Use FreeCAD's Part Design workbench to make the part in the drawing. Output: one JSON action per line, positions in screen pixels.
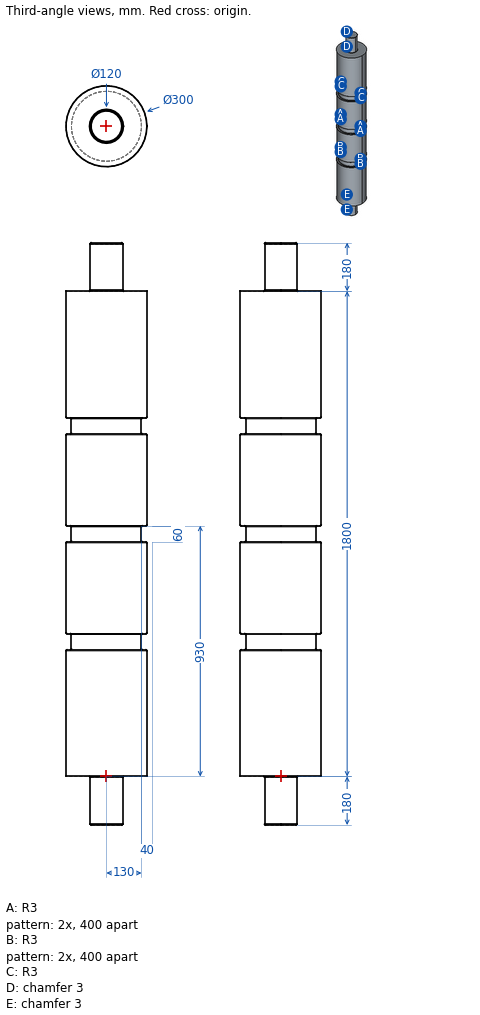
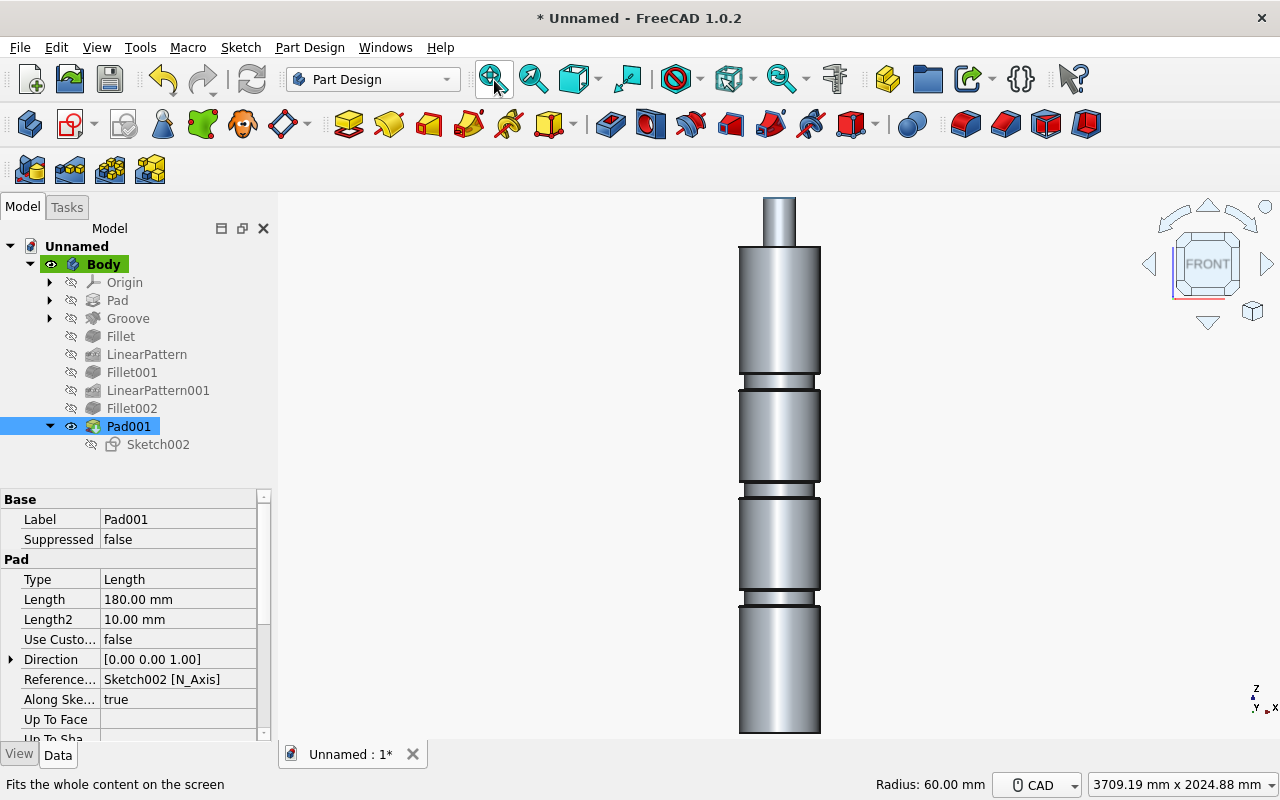
{"action": "key", "text": "3"}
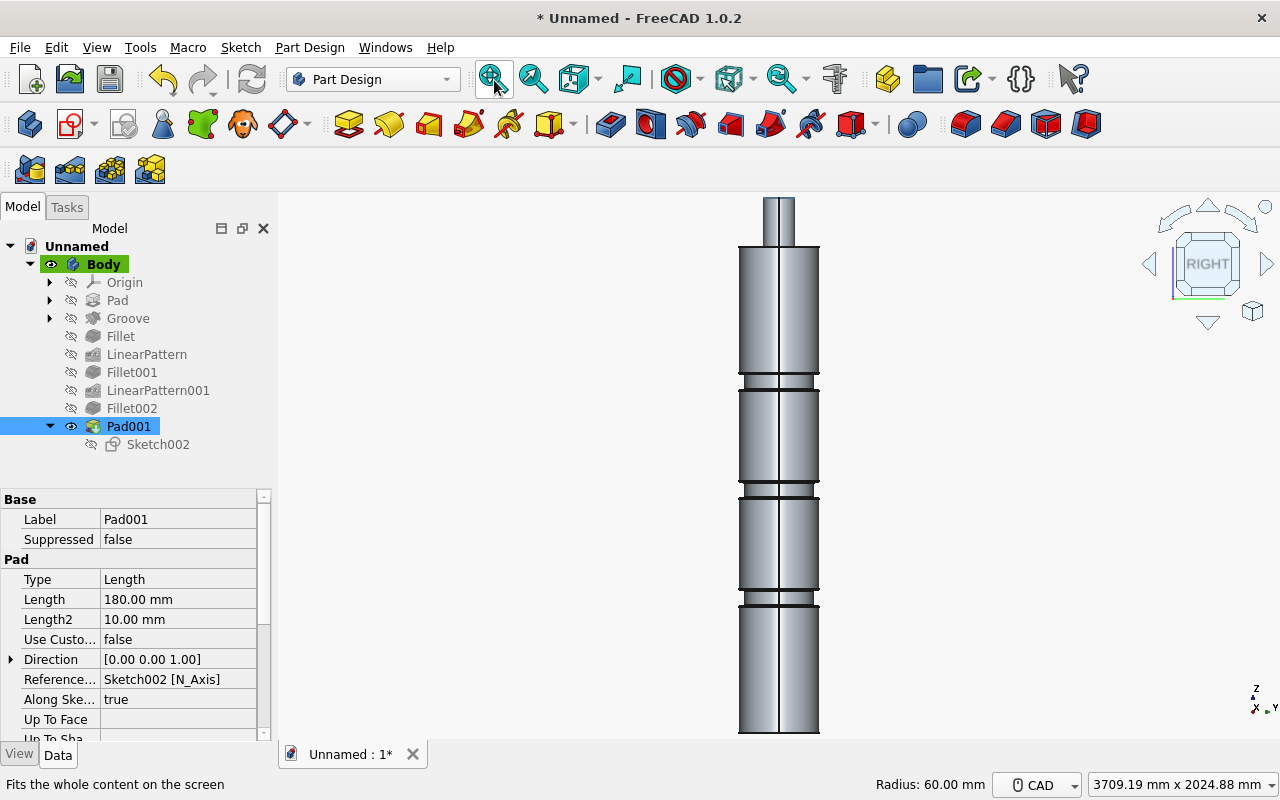
{"action": "key", "text": "5"}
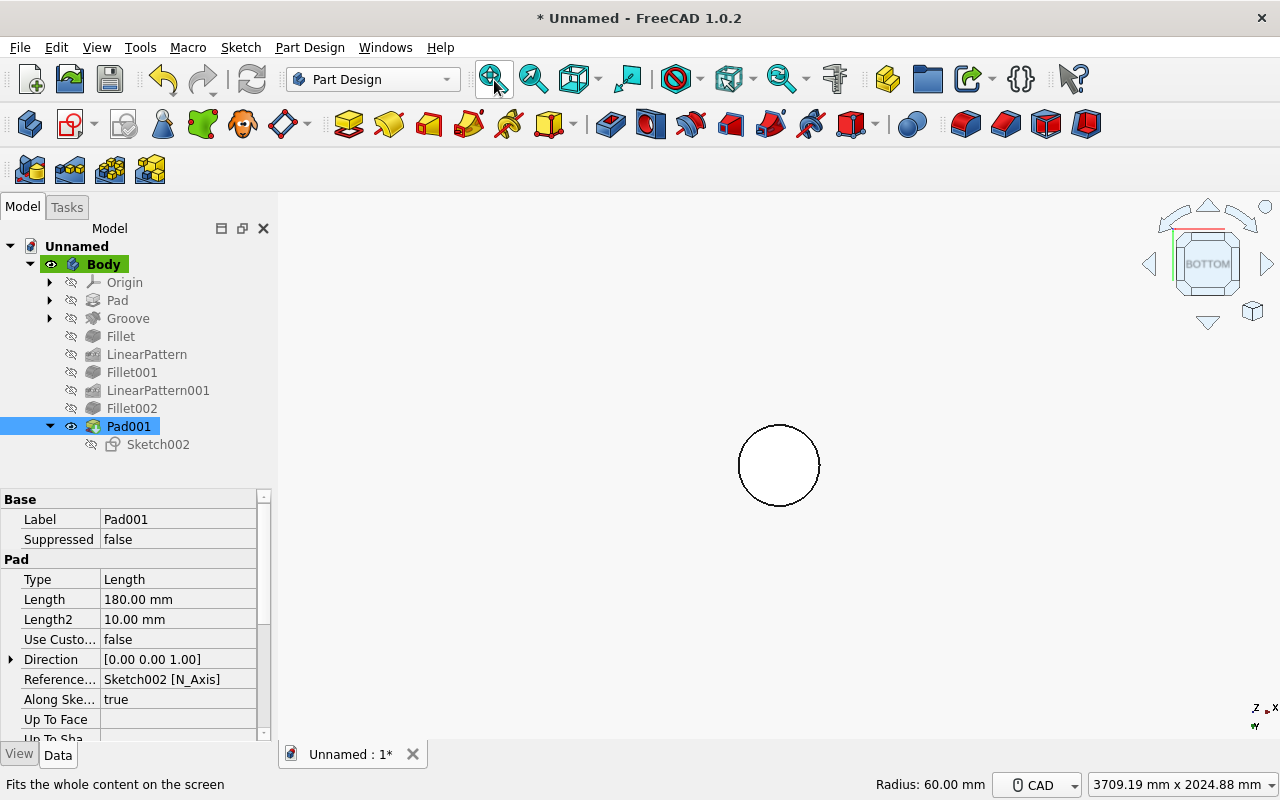
{"action": "left_click", "coordinate": [494, 80]}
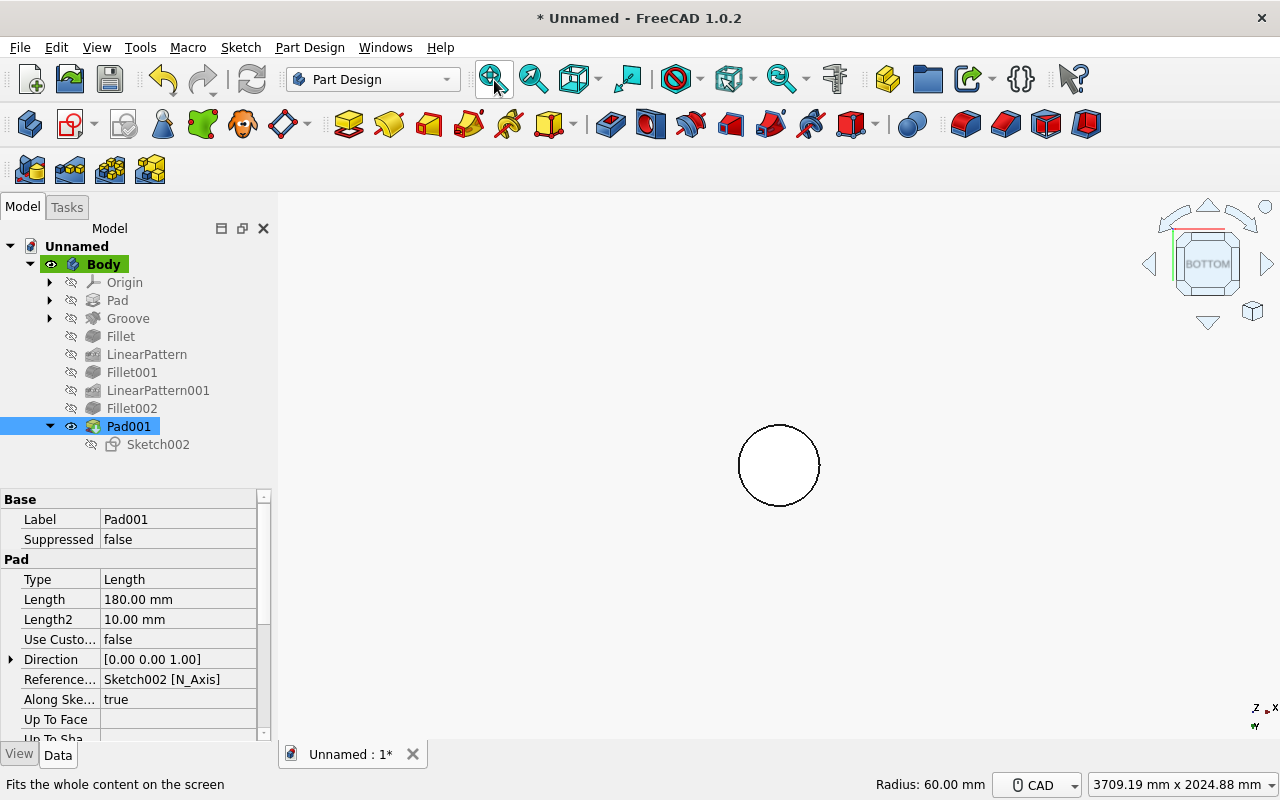
{"action": "key", "text": "4"}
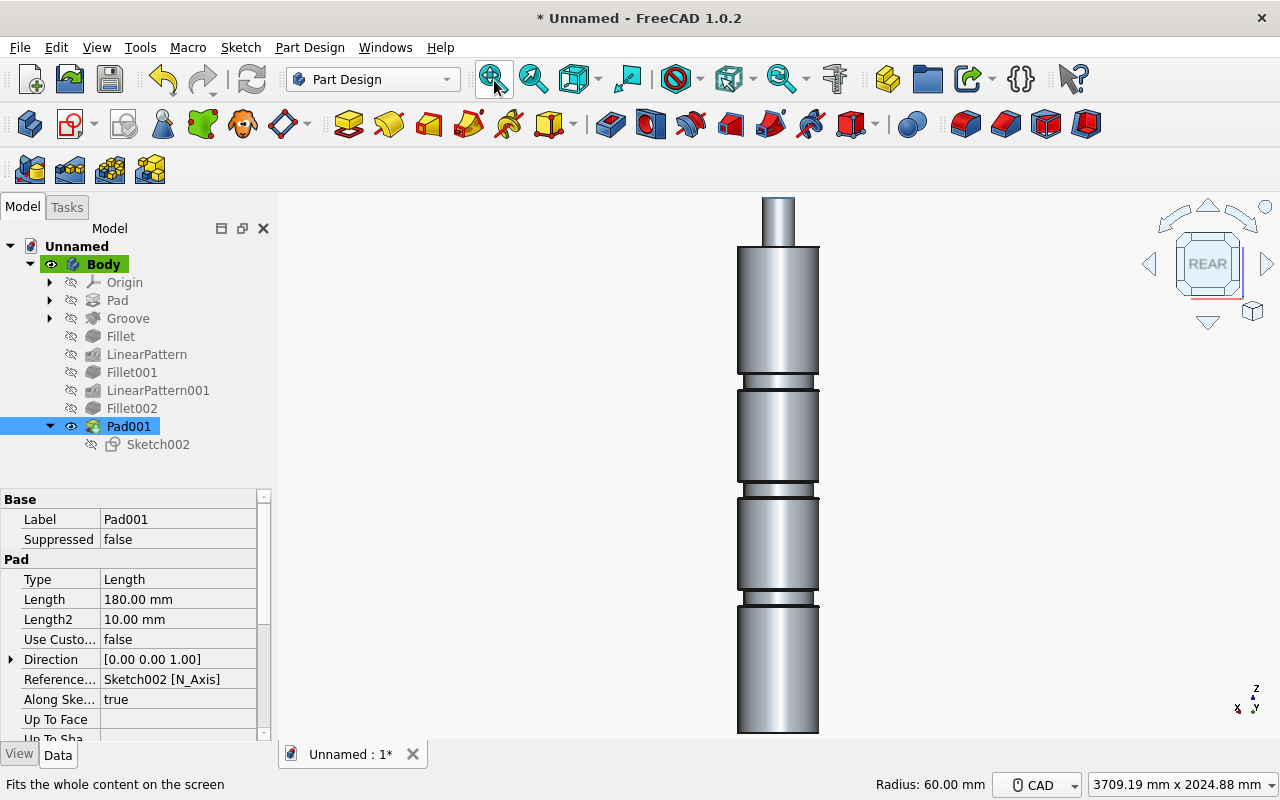
{"action": "key", "text": "6"}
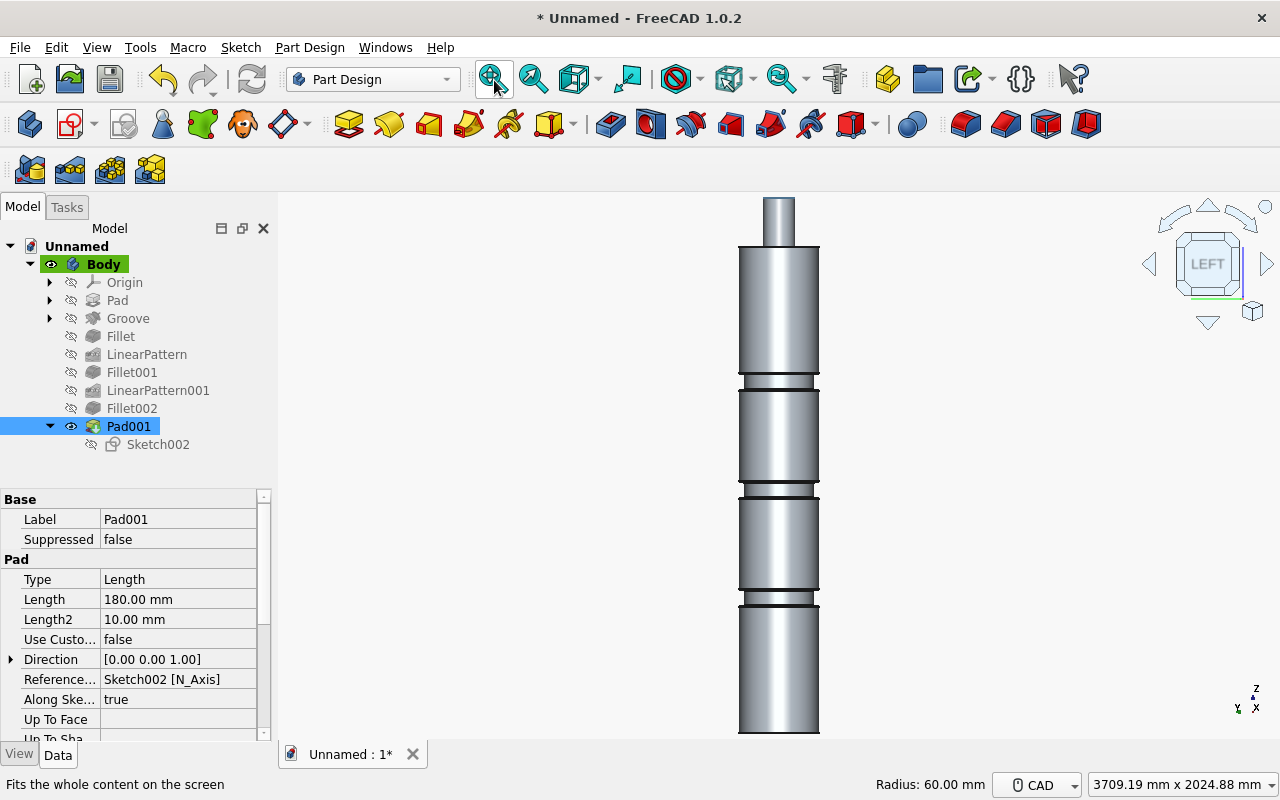
{"action": "key", "text": "v 3"}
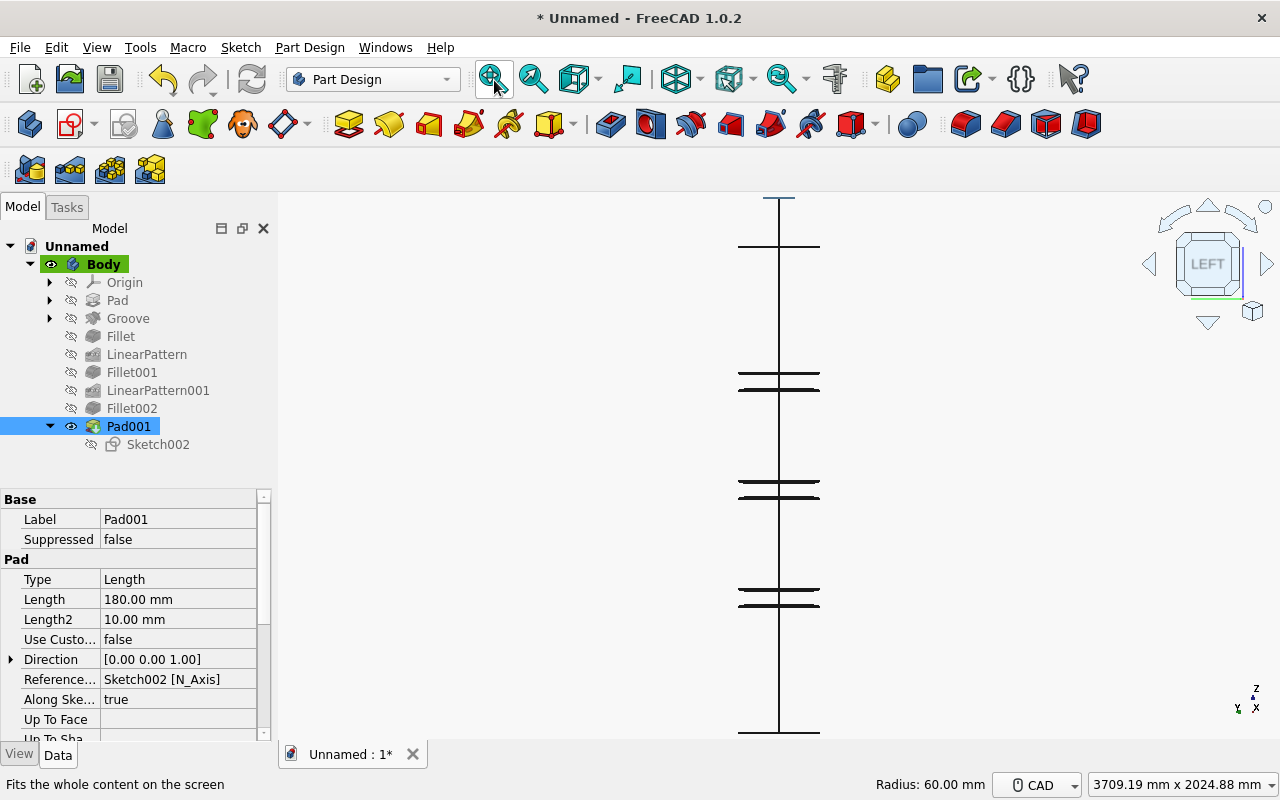
{"action": "key", "text": "0"}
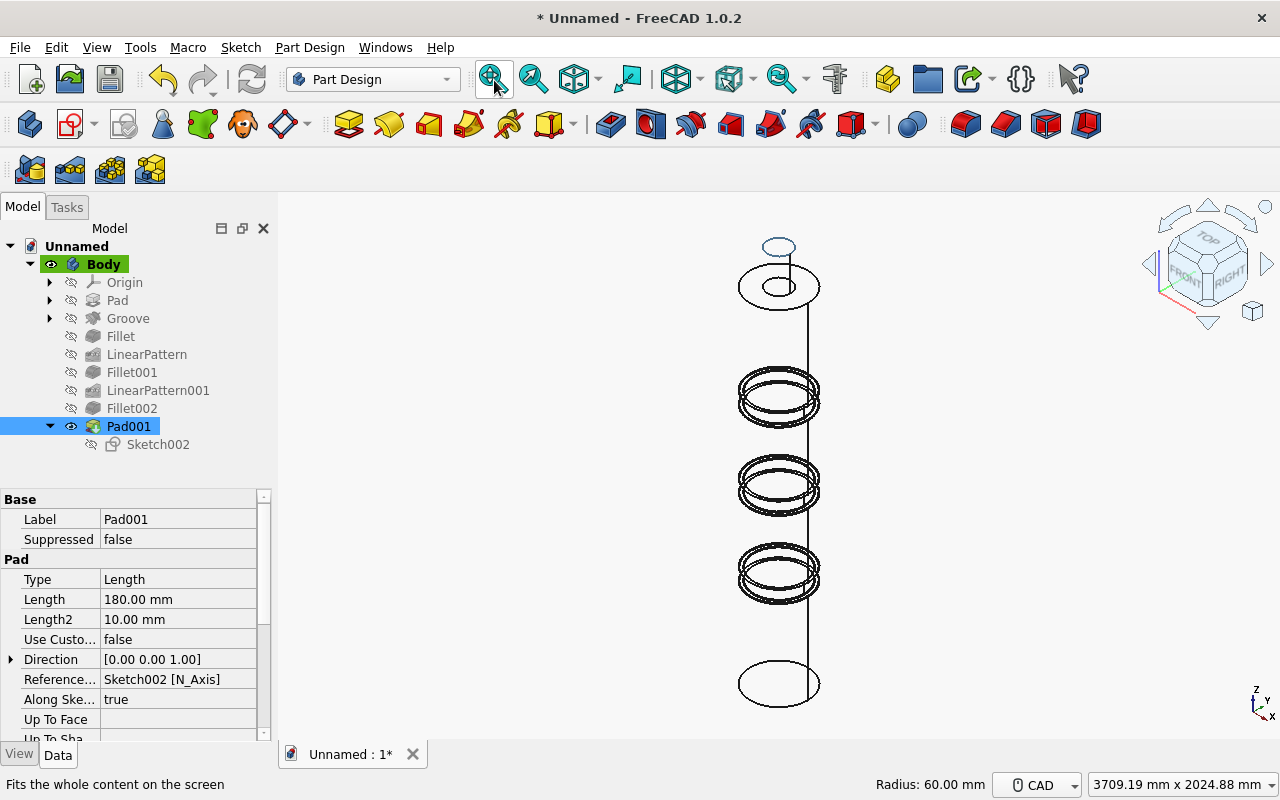
{"action": "left_click", "coordinate": [768, 279], "text": "ctrl"}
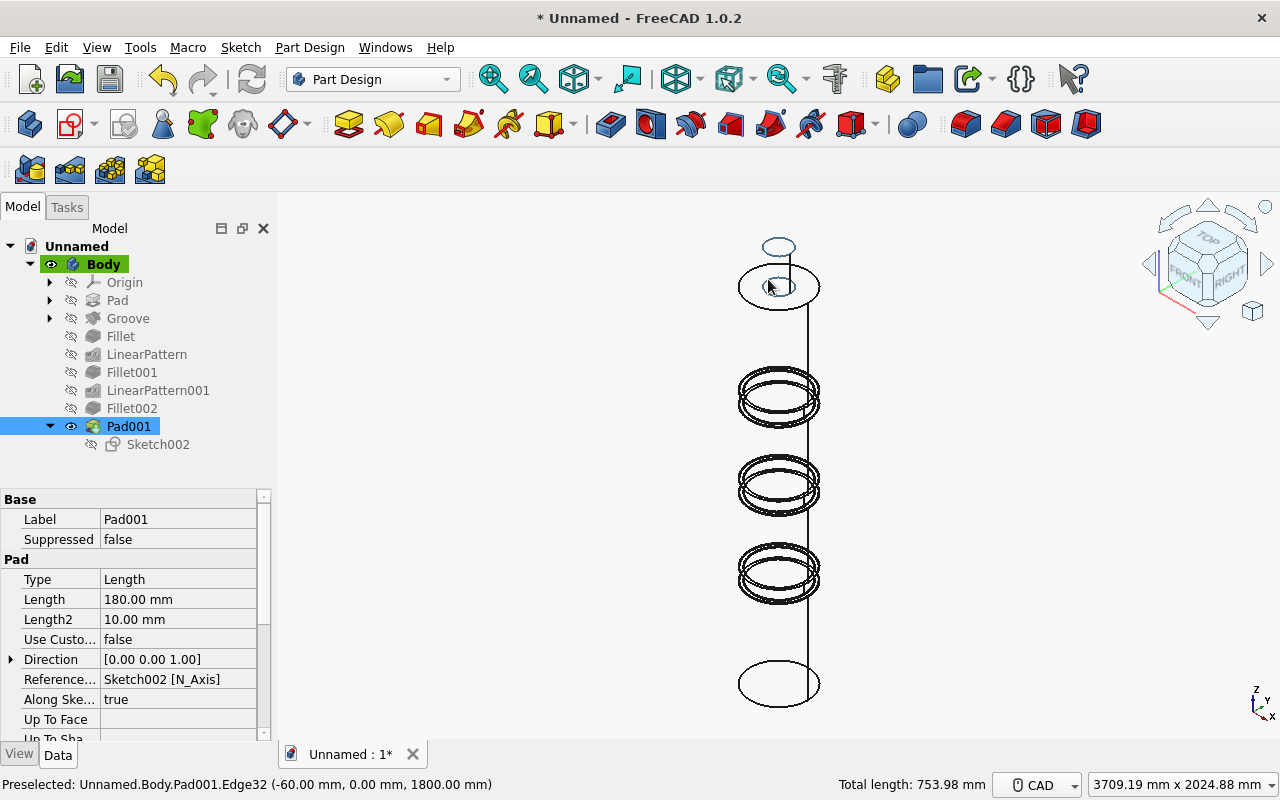
{"action": "key", "text": "v 1"}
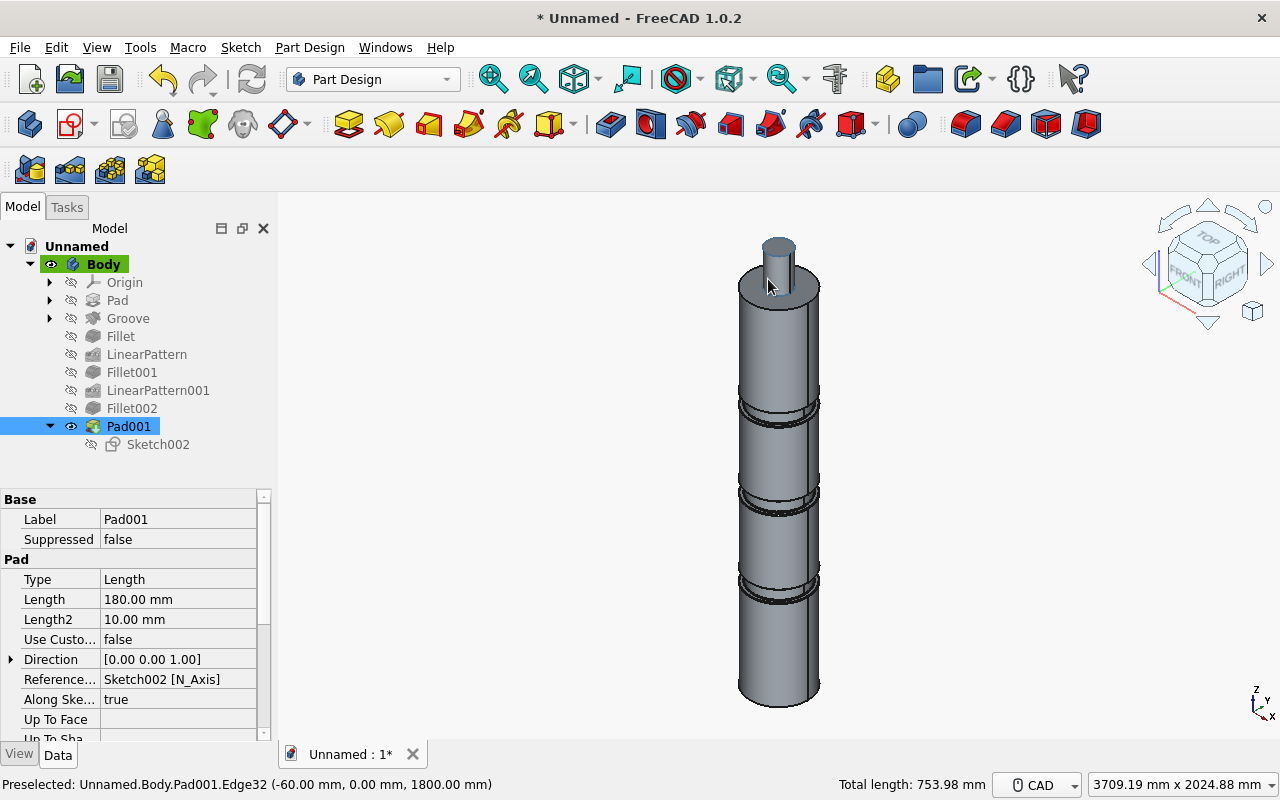
{"action": "left_click", "coordinate": [1006, 124]}